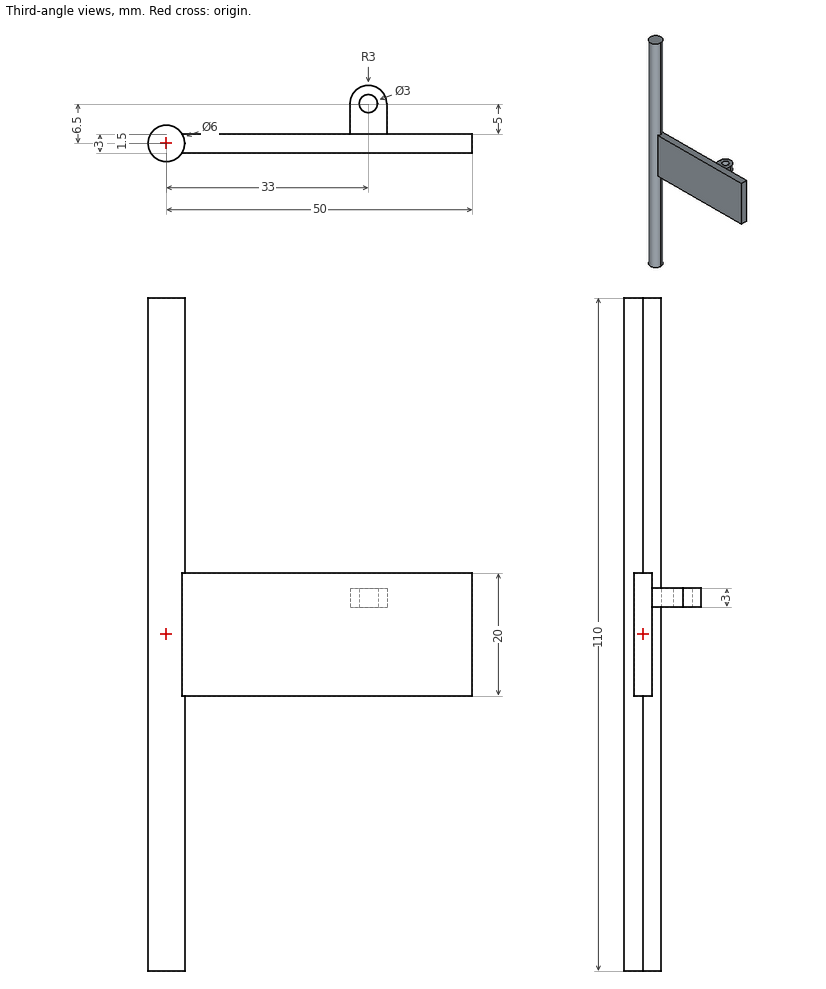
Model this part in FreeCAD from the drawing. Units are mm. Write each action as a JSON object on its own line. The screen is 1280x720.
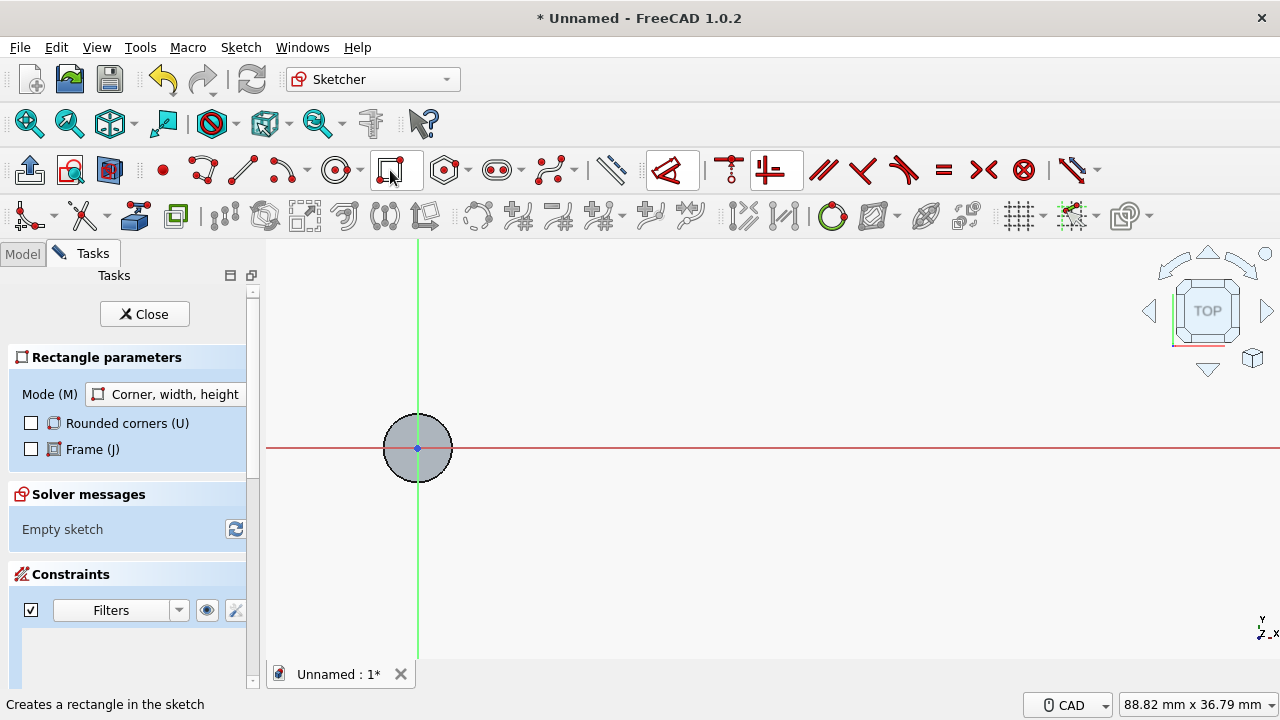
{"action": "left_click", "coordinate": [418, 431]}
{"action": "left_click", "coordinate": [989, 465]}
{"action": "key", "text": "Escape"}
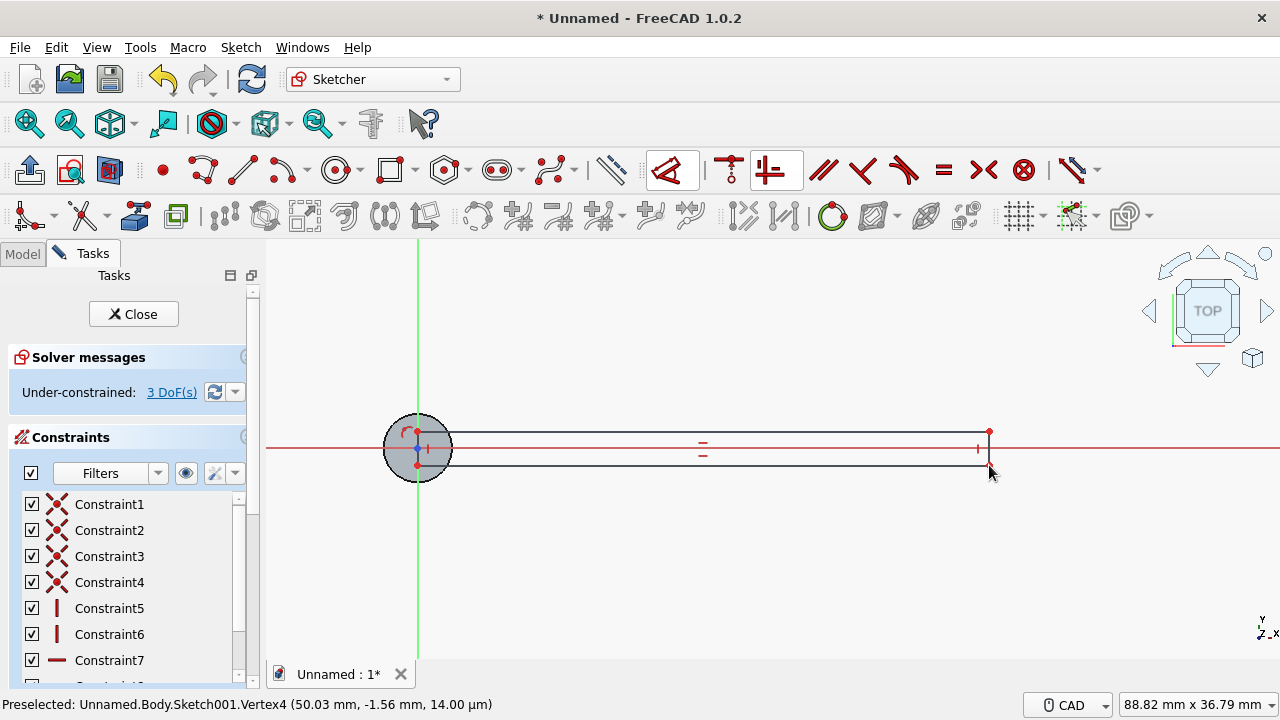
{"action": "left_click", "coordinate": [418, 456]}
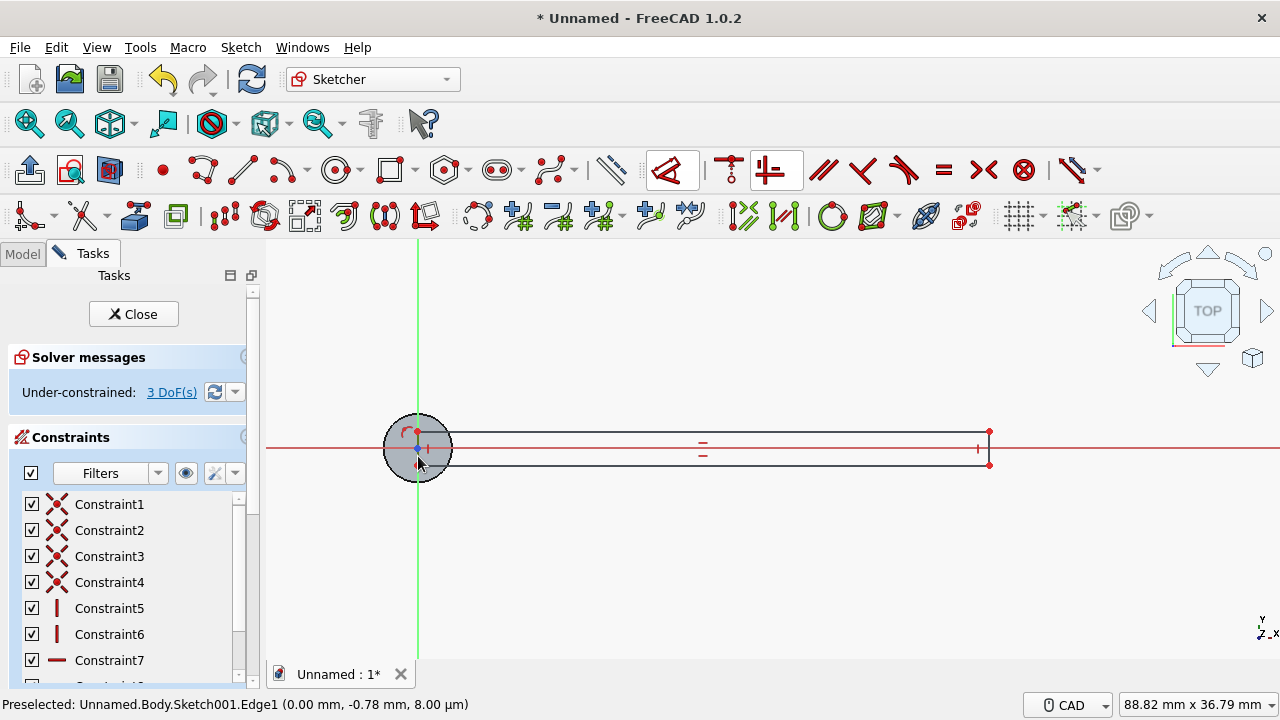
{"action": "left_click", "coordinate": [694, 170]}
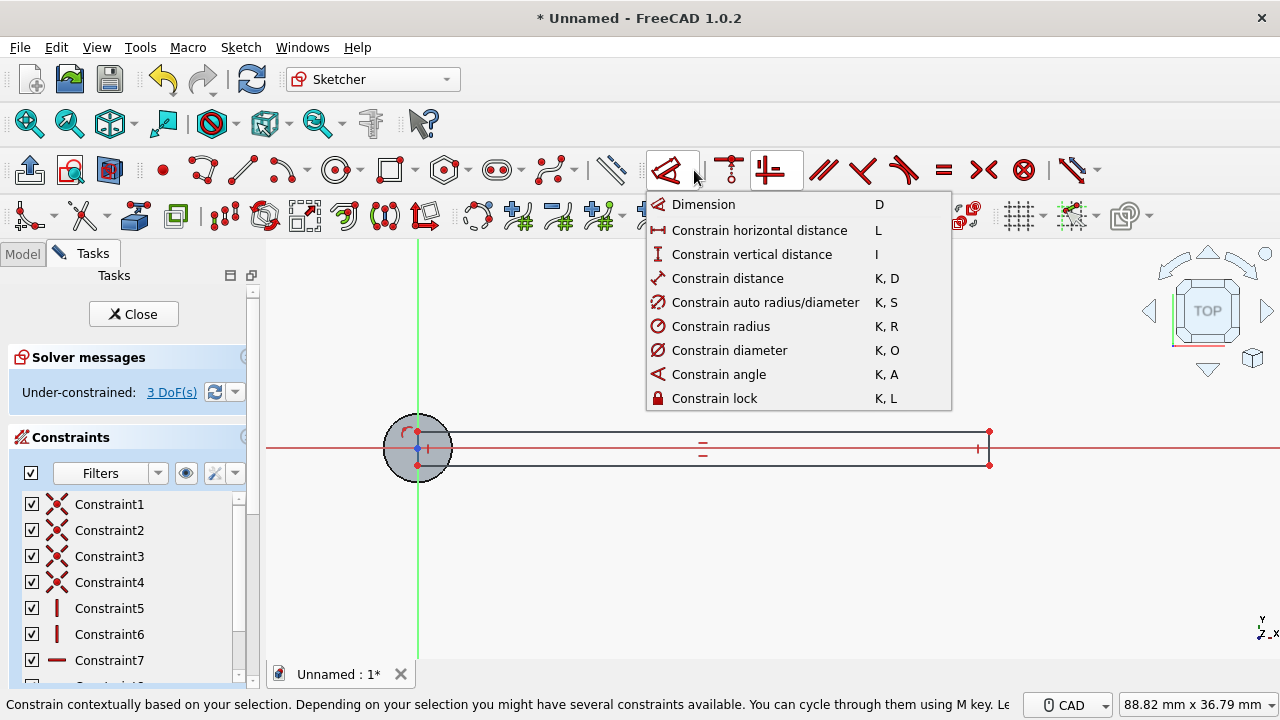
{"action": "left_click", "coordinate": [799, 254]}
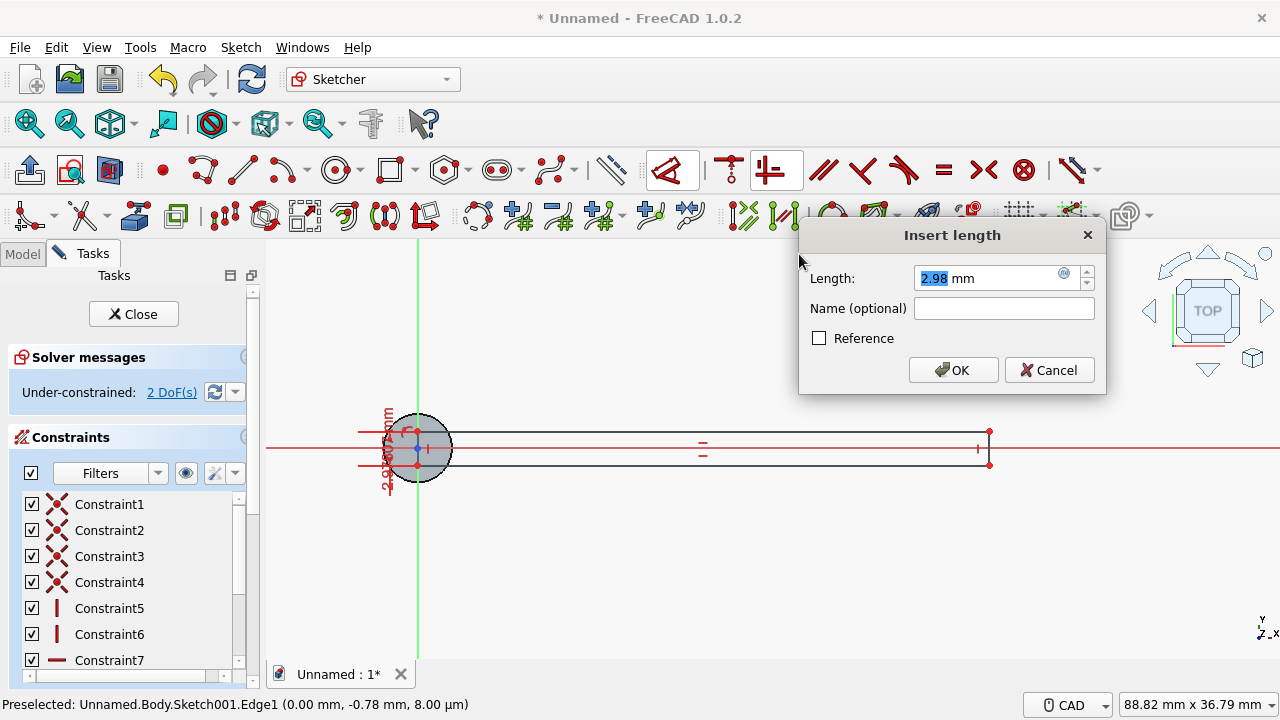
{"action": "type", "text": "3"}
{"action": "key", "text": "Return"}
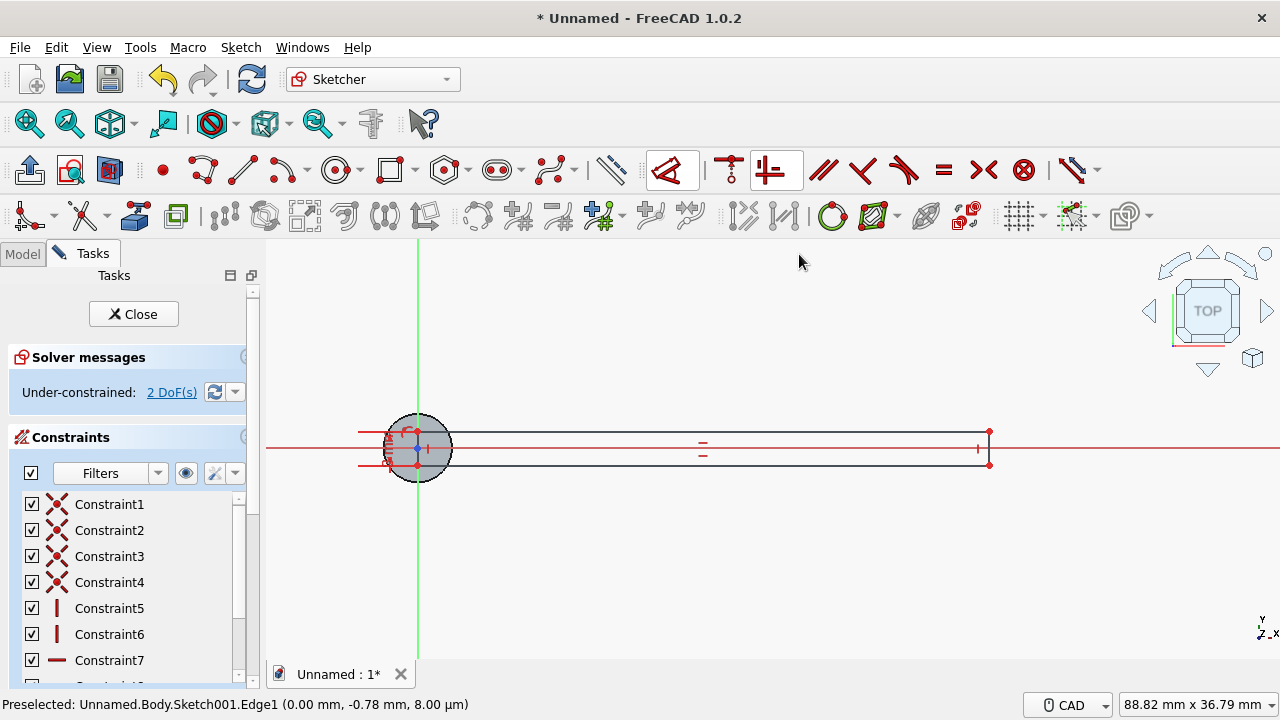
{"action": "left_click", "coordinate": [589, 466]}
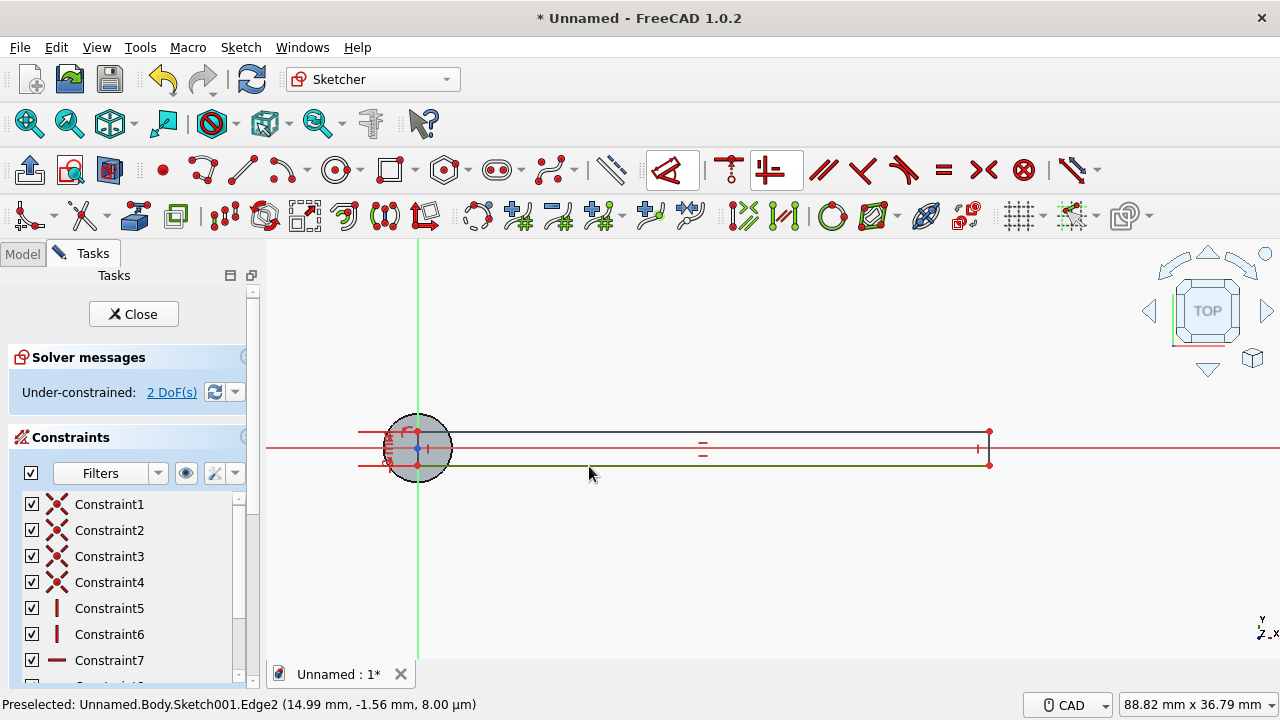
{"action": "left_click", "coordinate": [694, 170]}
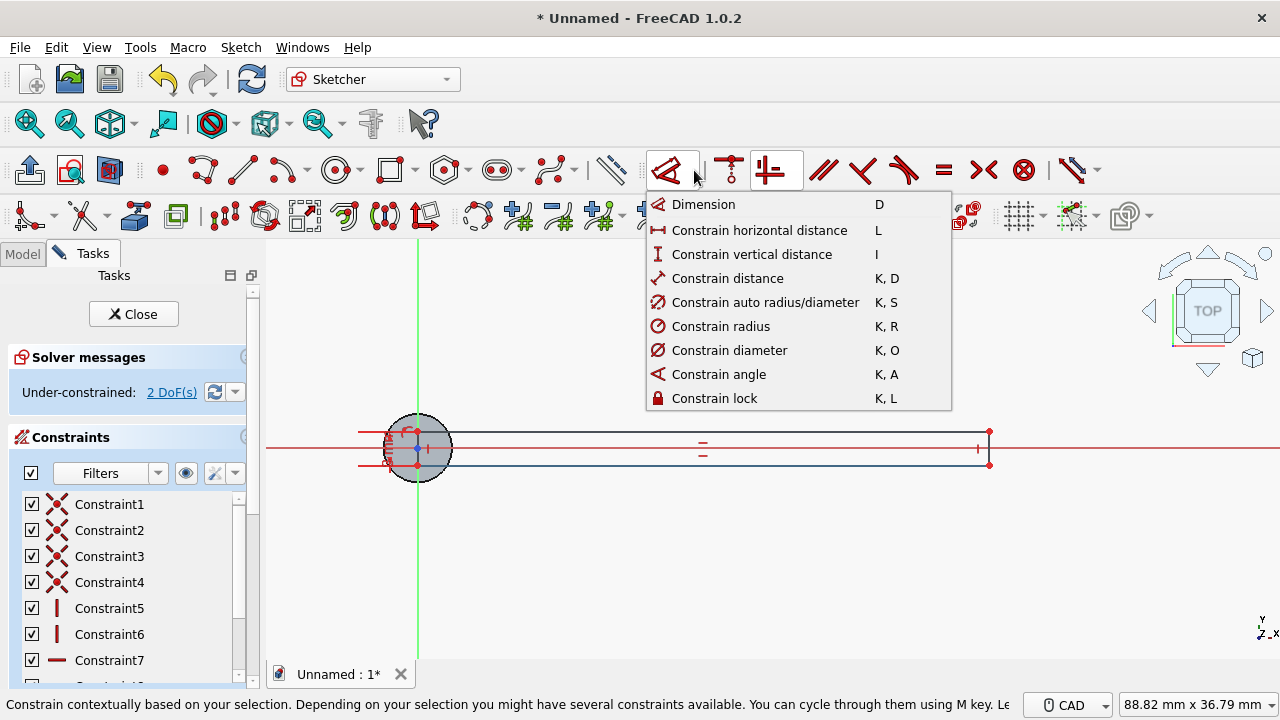
{"action": "left_click", "coordinate": [799, 230]}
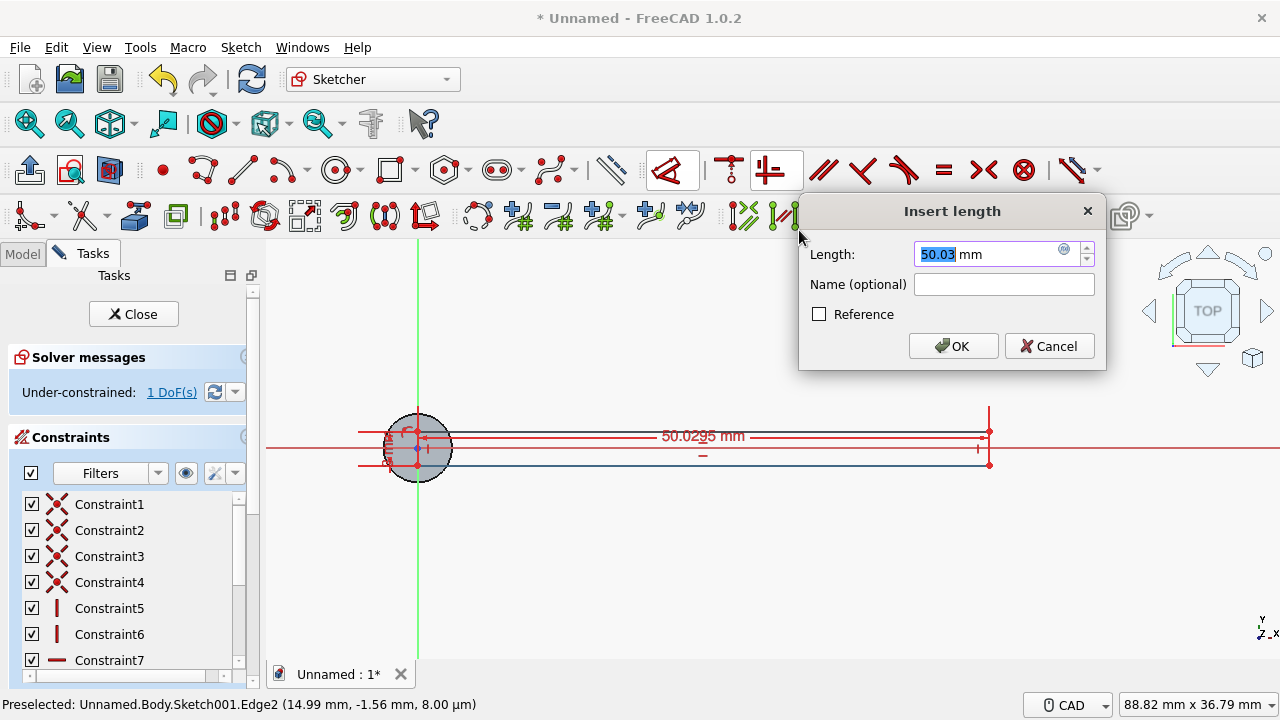
{"action": "type", "text": "50"}
{"action": "key", "text": "Return"}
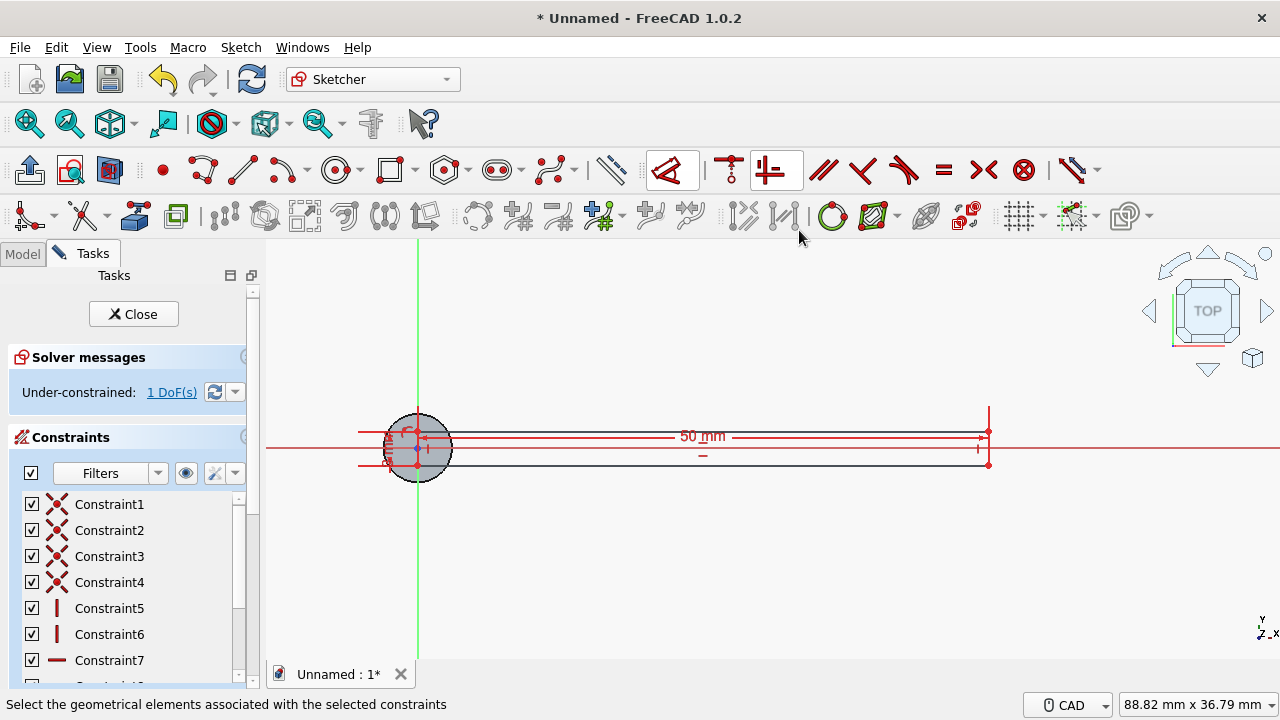
{"action": "scroll", "coordinate": [418, 432], "scroll_direction": "up", "scroll_amount": 5}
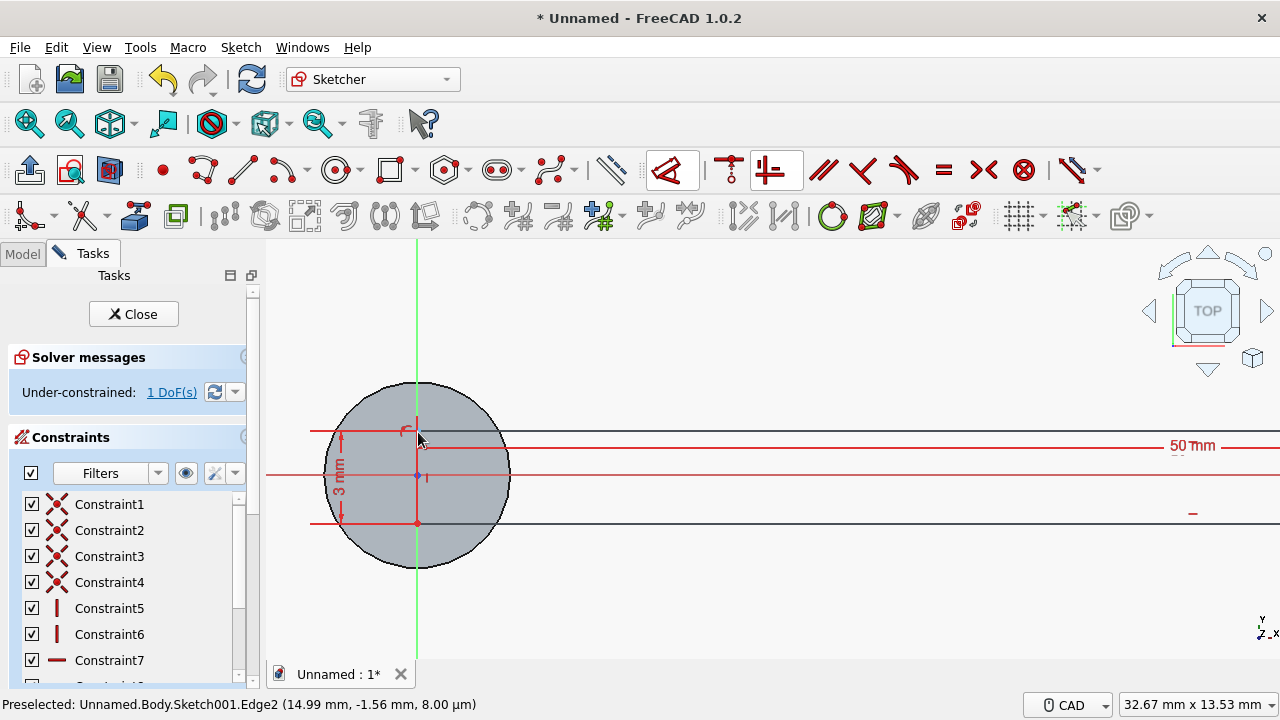
{"action": "left_click", "coordinate": [417, 431]}